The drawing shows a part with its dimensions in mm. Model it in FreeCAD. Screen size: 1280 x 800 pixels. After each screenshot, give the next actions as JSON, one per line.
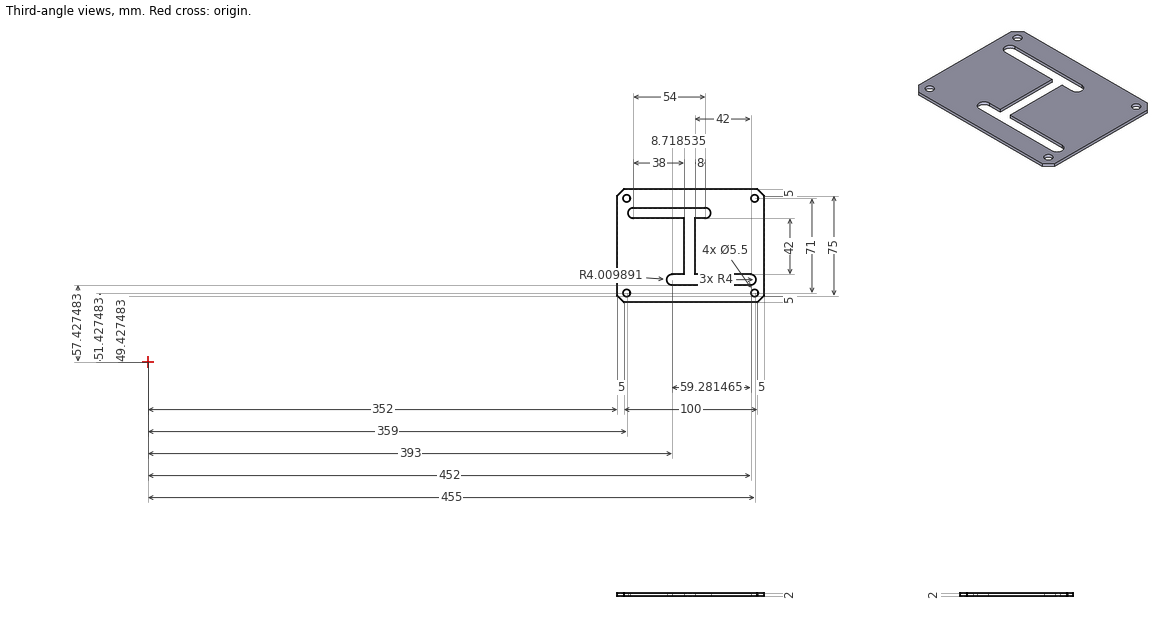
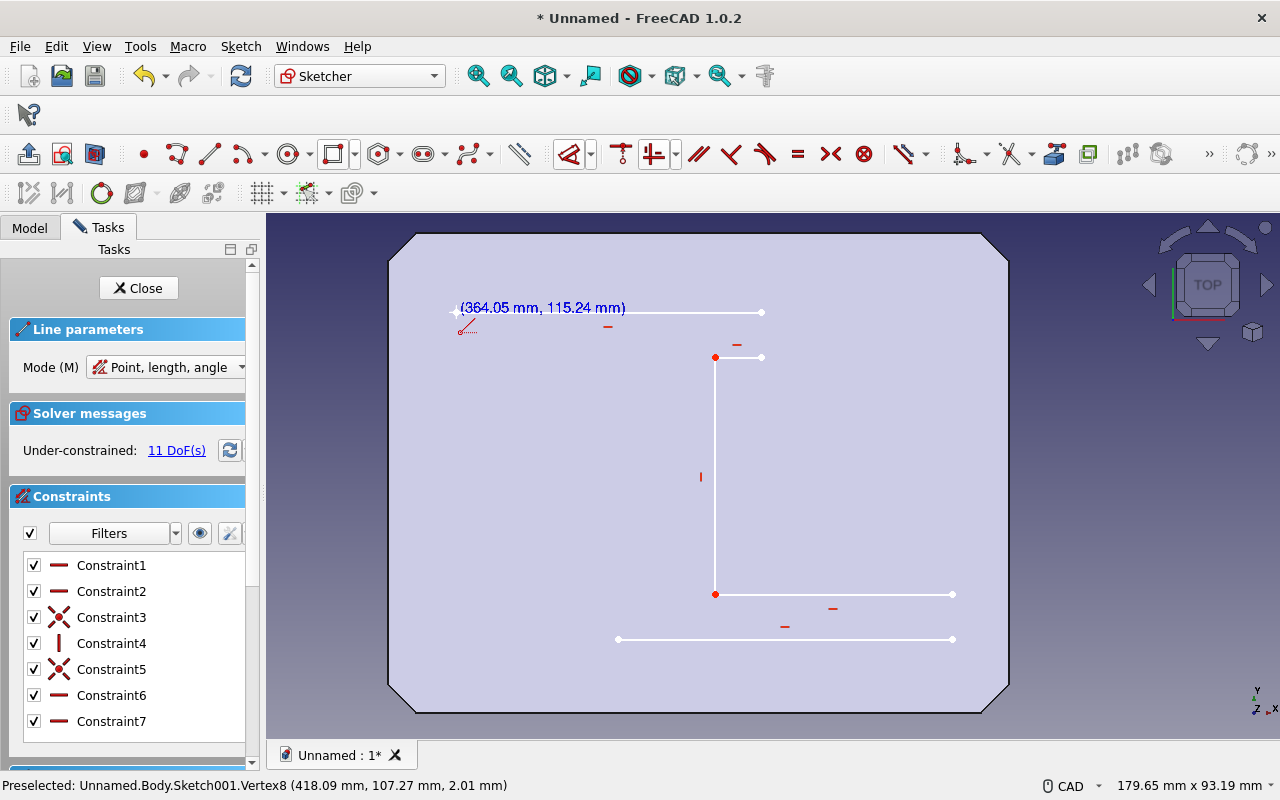
{"action": "left_click", "coordinate": [177, 154]}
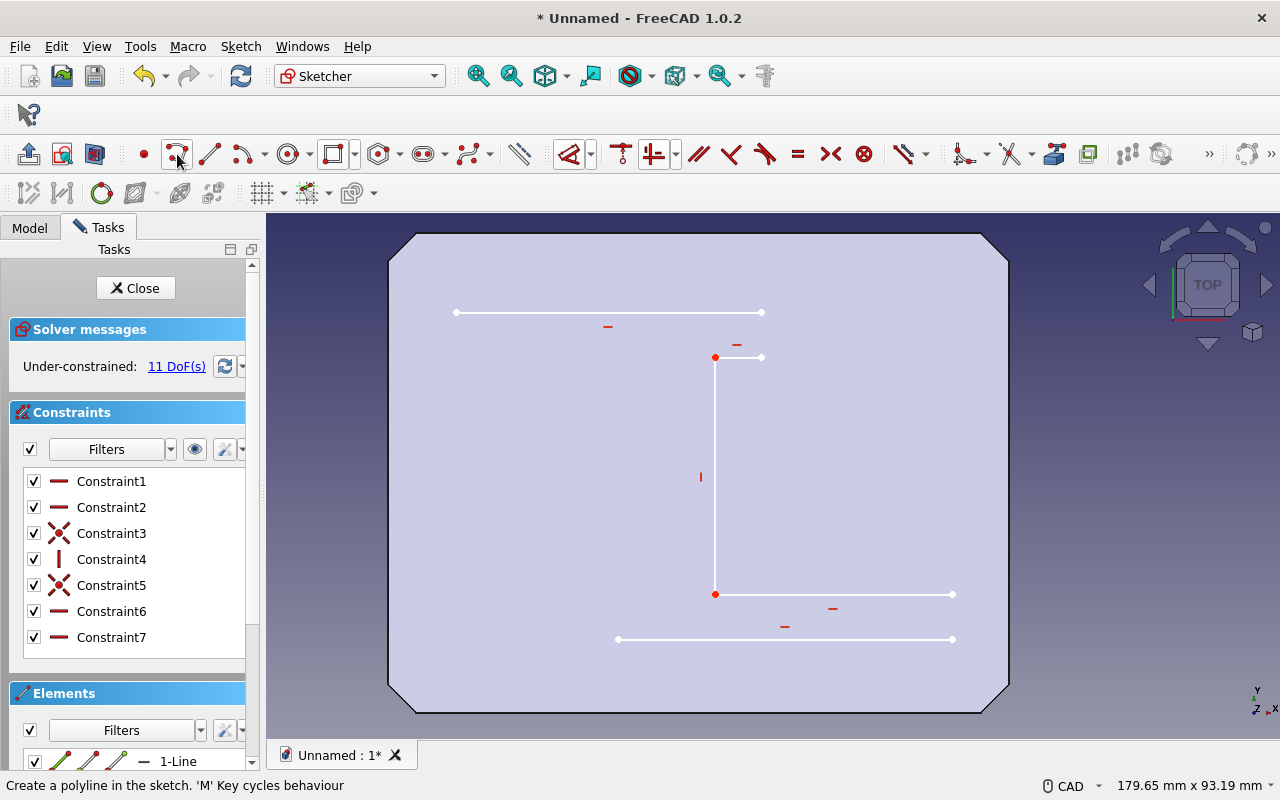
{"action": "left_click", "coordinate": [456, 357]}
{"action": "left_click", "coordinate": [670, 357]}
{"action": "left_click", "coordinate": [670, 594]}
{"action": "left_click", "coordinate": [621, 594]}
{"action": "right_click", "coordinate": [621, 594]}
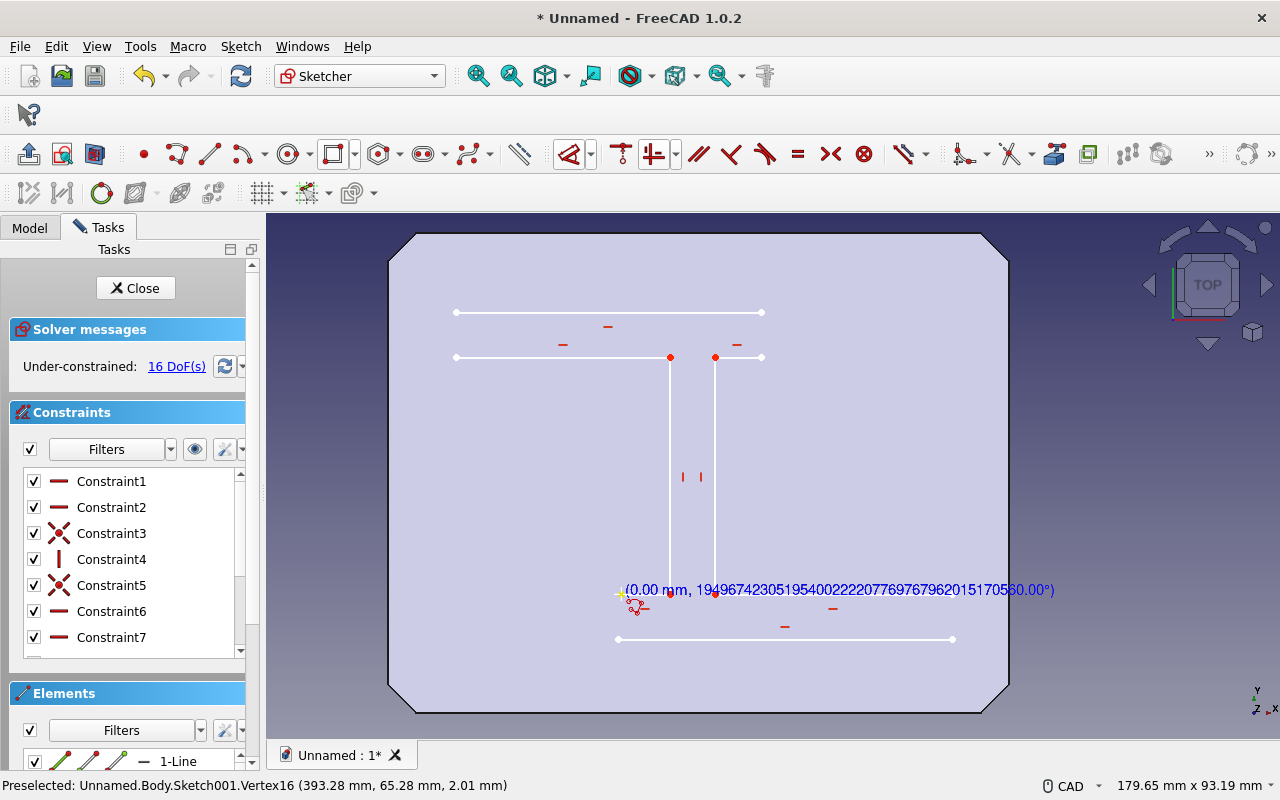
{"action": "left_click", "coordinate": [264, 154]}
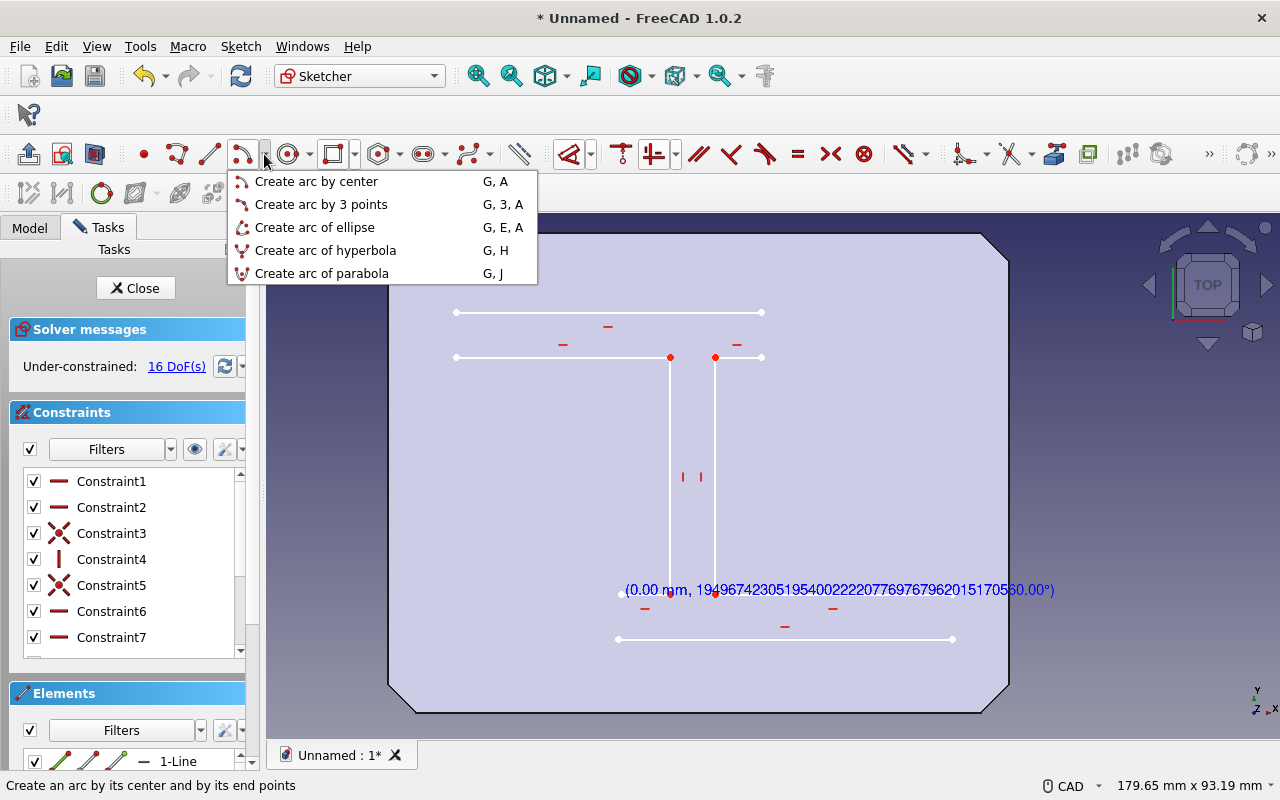
{"action": "left_click", "coordinate": [382, 204]}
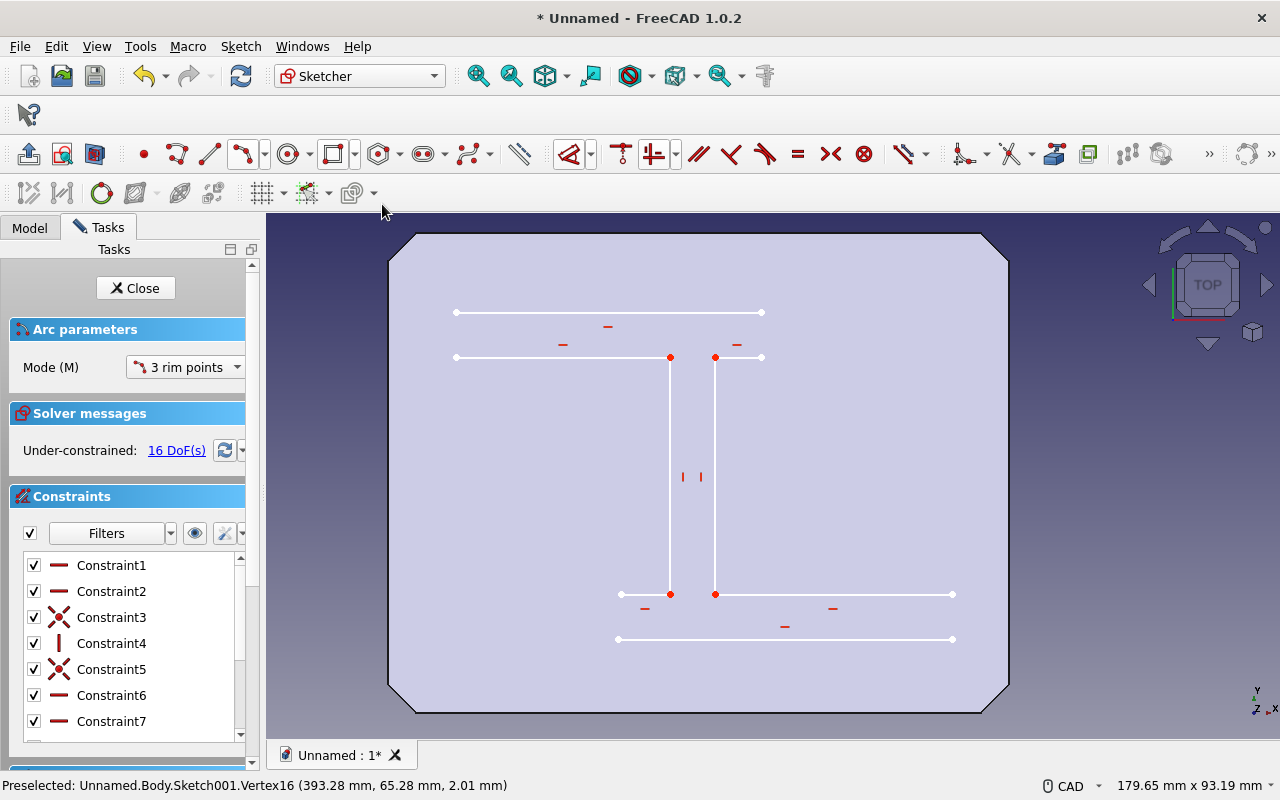
{"action": "left_click", "coordinate": [952, 640]}
{"action": "left_click", "coordinate": [952, 595]}
{"action": "left_click", "coordinate": [975, 617]}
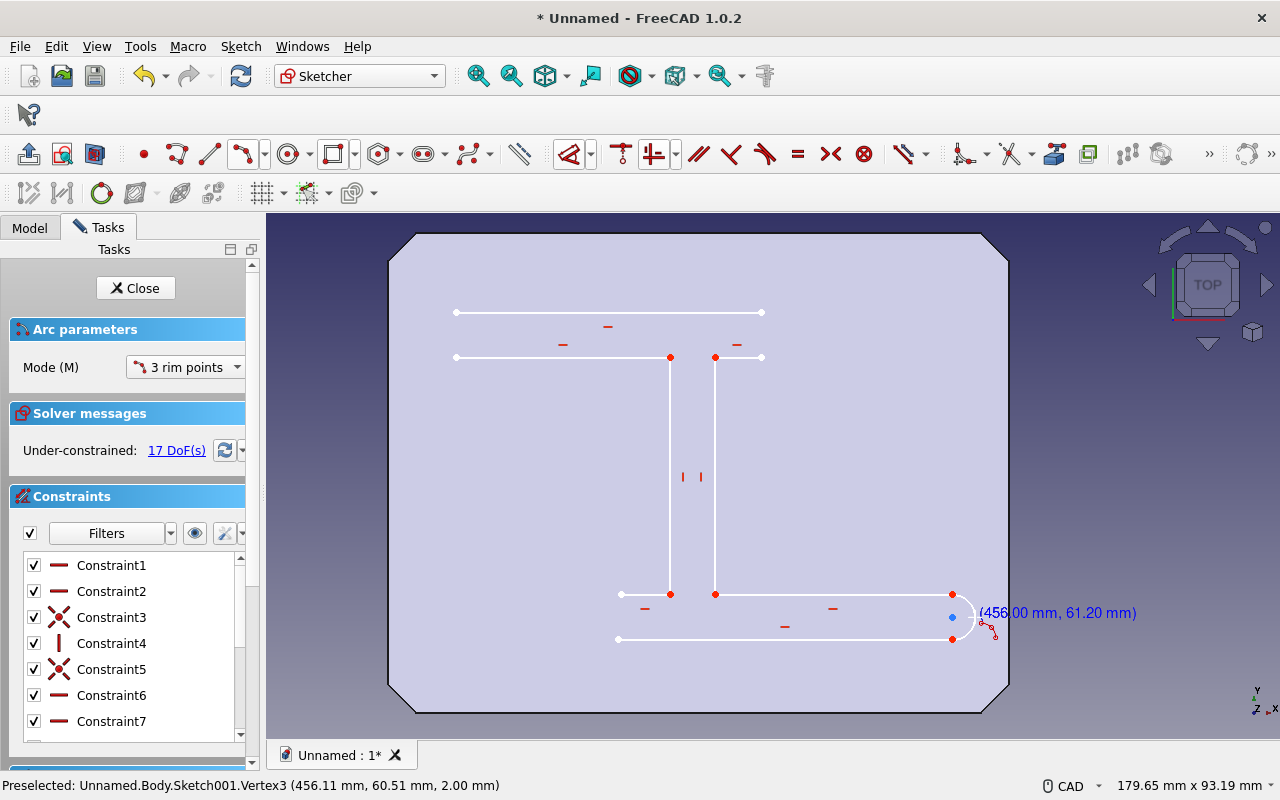
{"action": "left_click", "coordinate": [761, 358]}
{"action": "left_click", "coordinate": [761, 313]}
{"action": "left_click", "coordinate": [783, 335]}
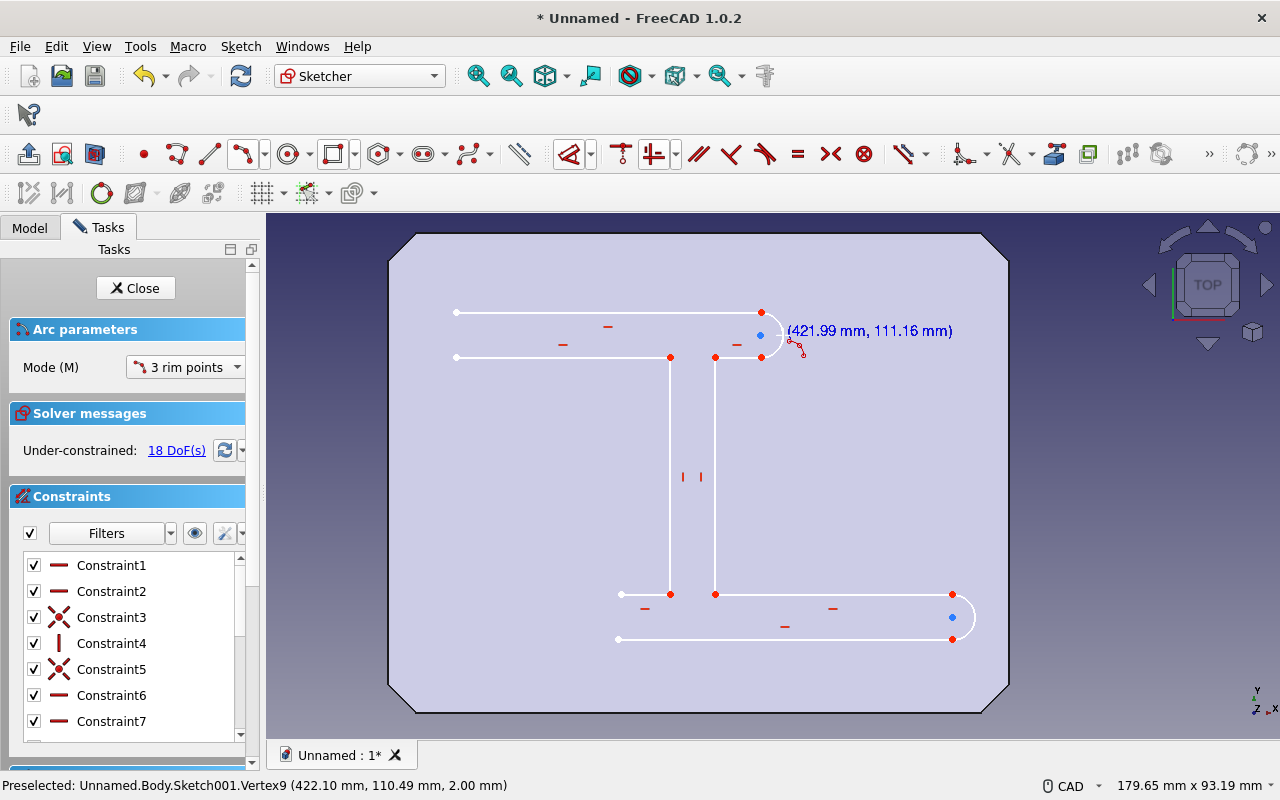
{"action": "left_click", "coordinate": [456, 313]}
{"action": "left_click", "coordinate": [456, 358]}
{"action": "left_click", "coordinate": [433, 335]}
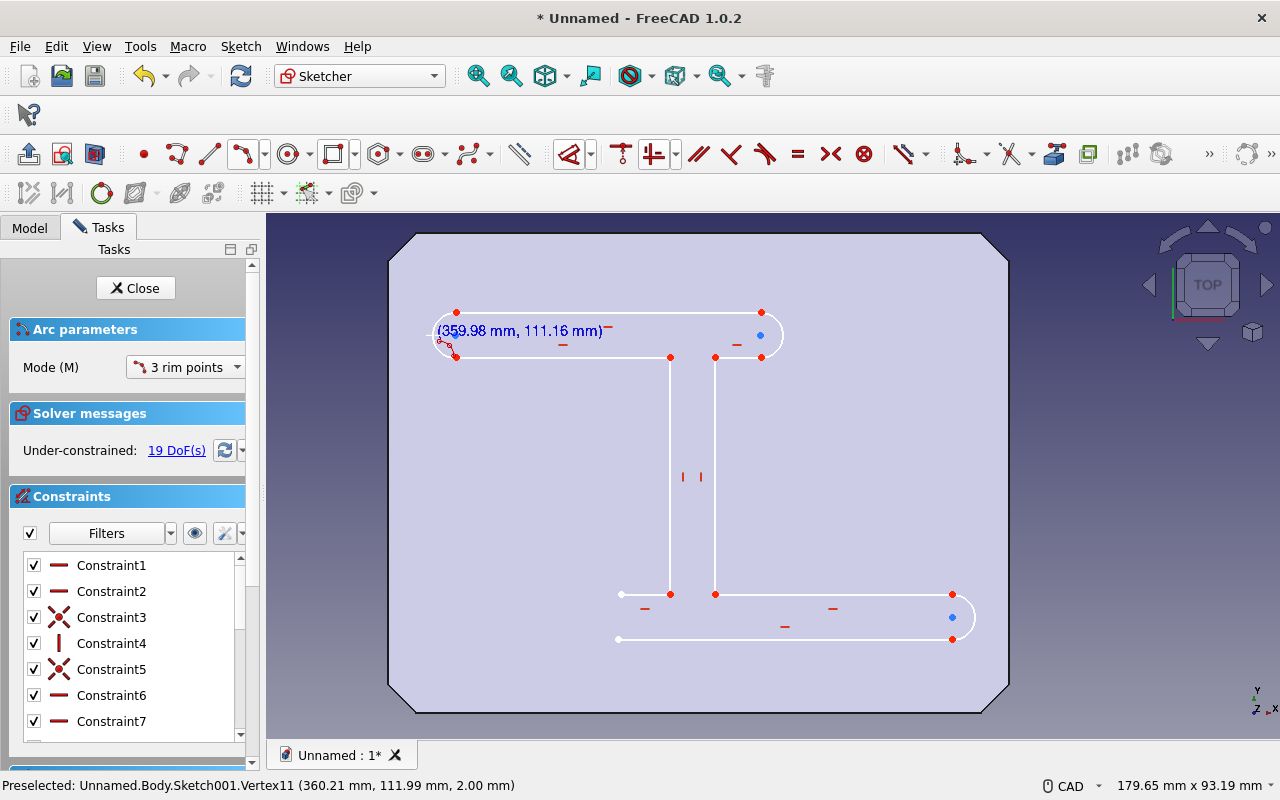
{"action": "left_click", "coordinate": [621, 595]}
{"action": "left_click", "coordinate": [618, 640]}
{"action": "left_click", "coordinate": [597, 615]}
{"action": "key", "text": "Escape"}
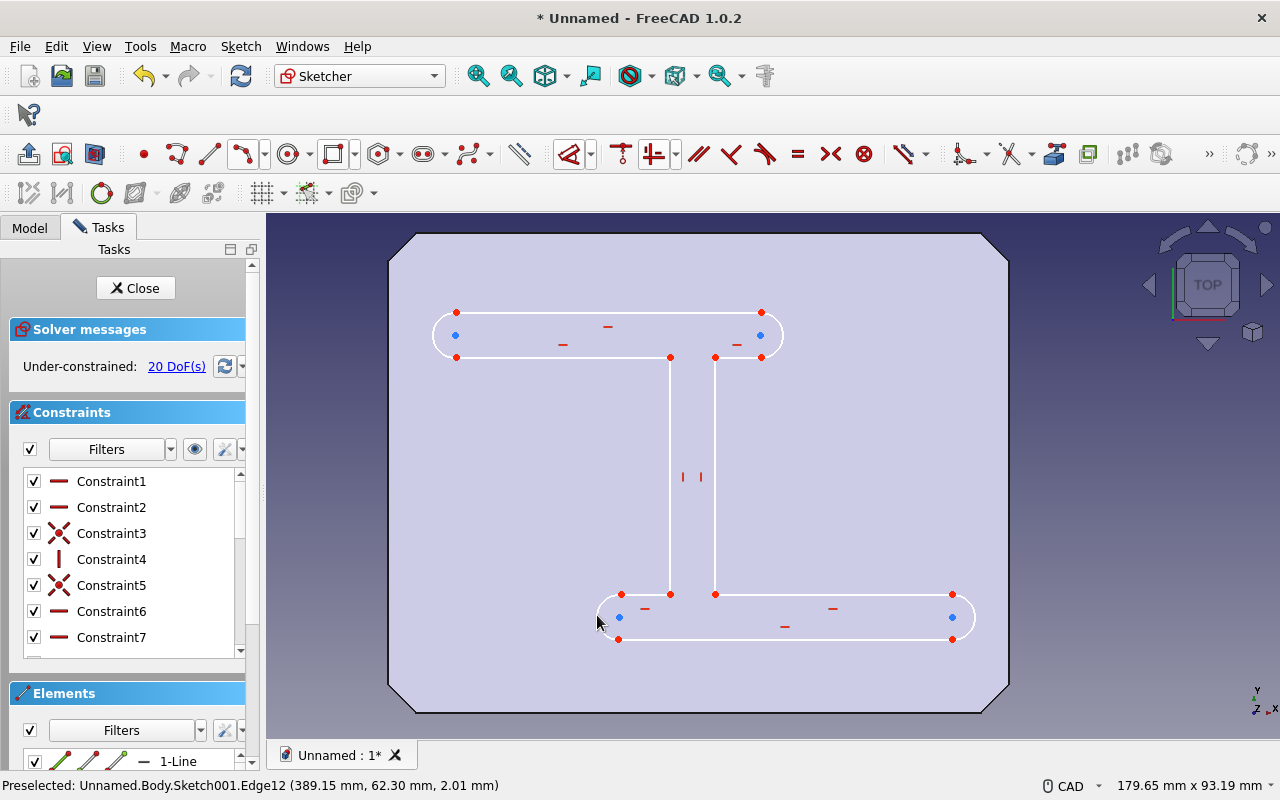
{"action": "left_click", "coordinate": [718, 640]}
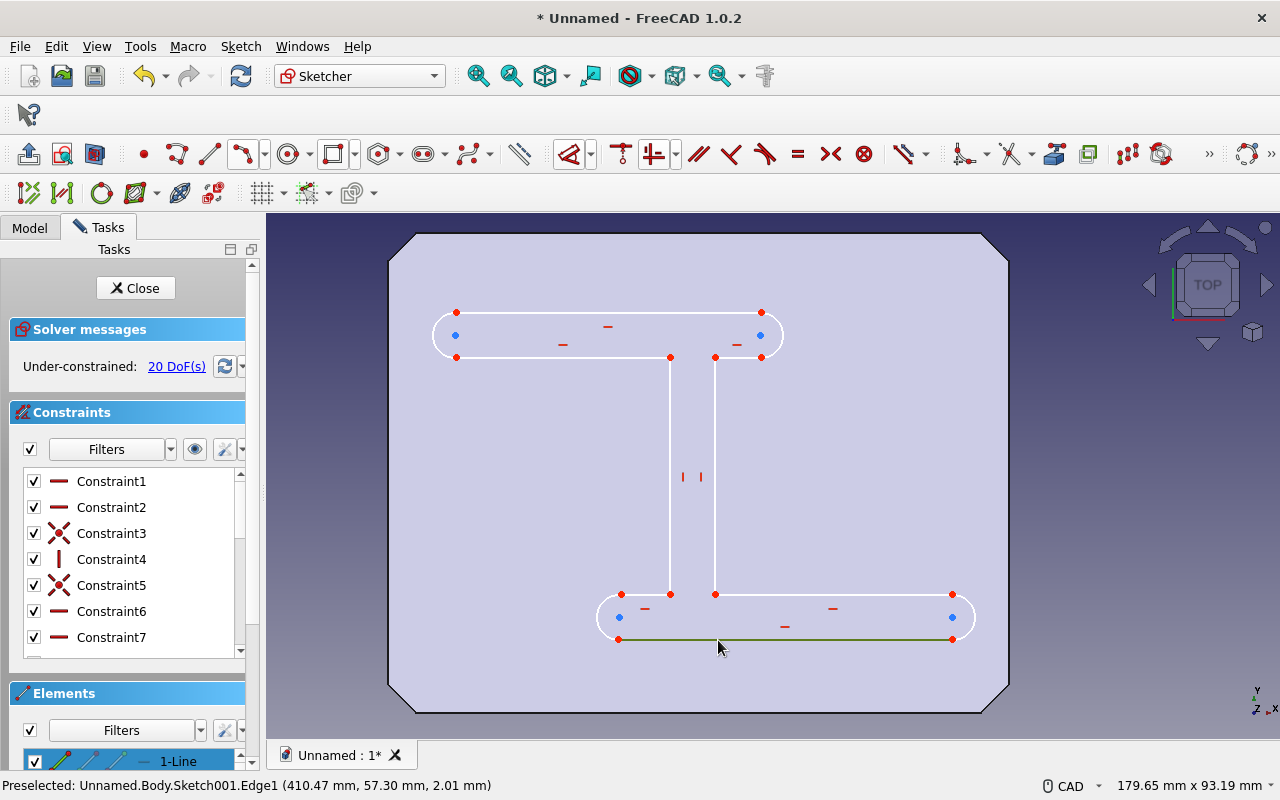
{"action": "left_click", "coordinate": [971, 631]}